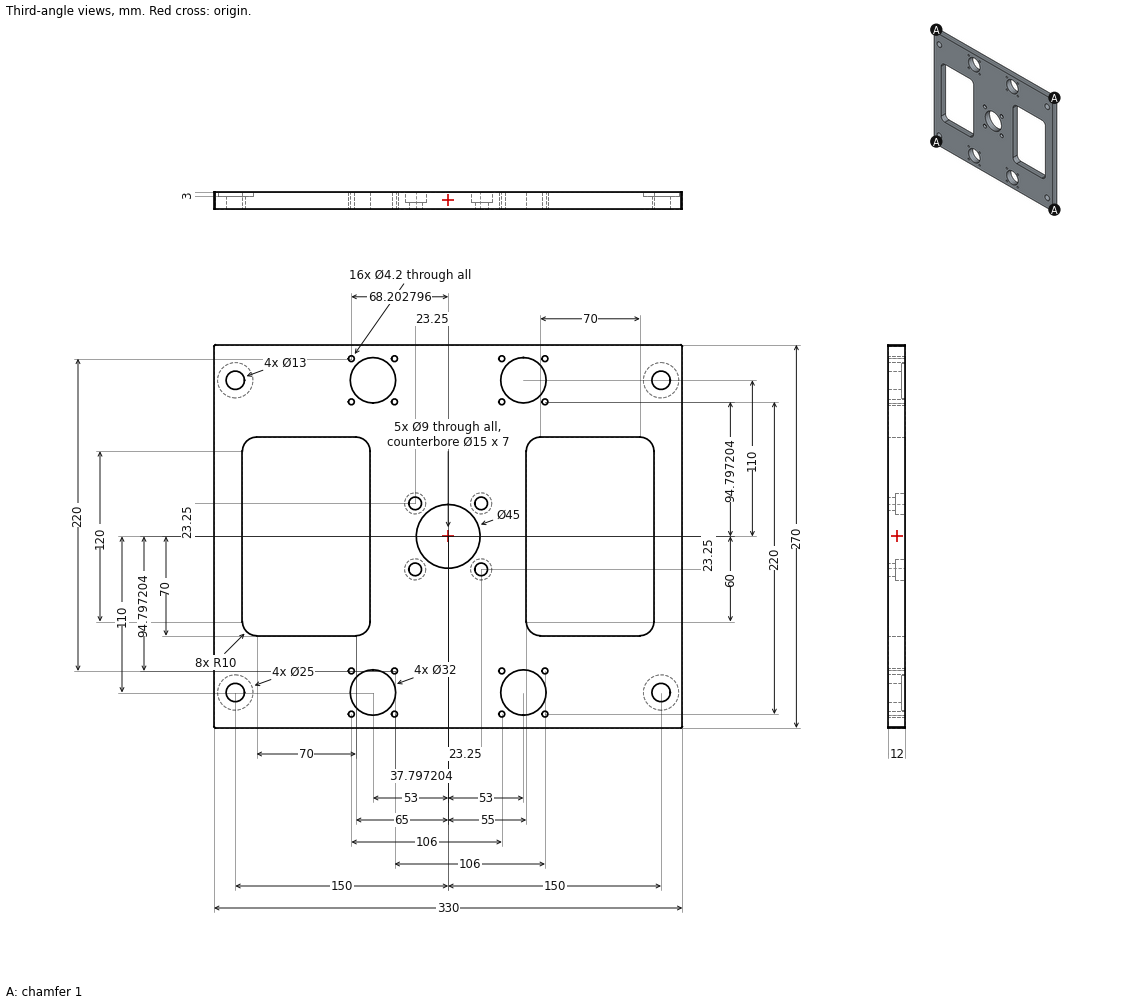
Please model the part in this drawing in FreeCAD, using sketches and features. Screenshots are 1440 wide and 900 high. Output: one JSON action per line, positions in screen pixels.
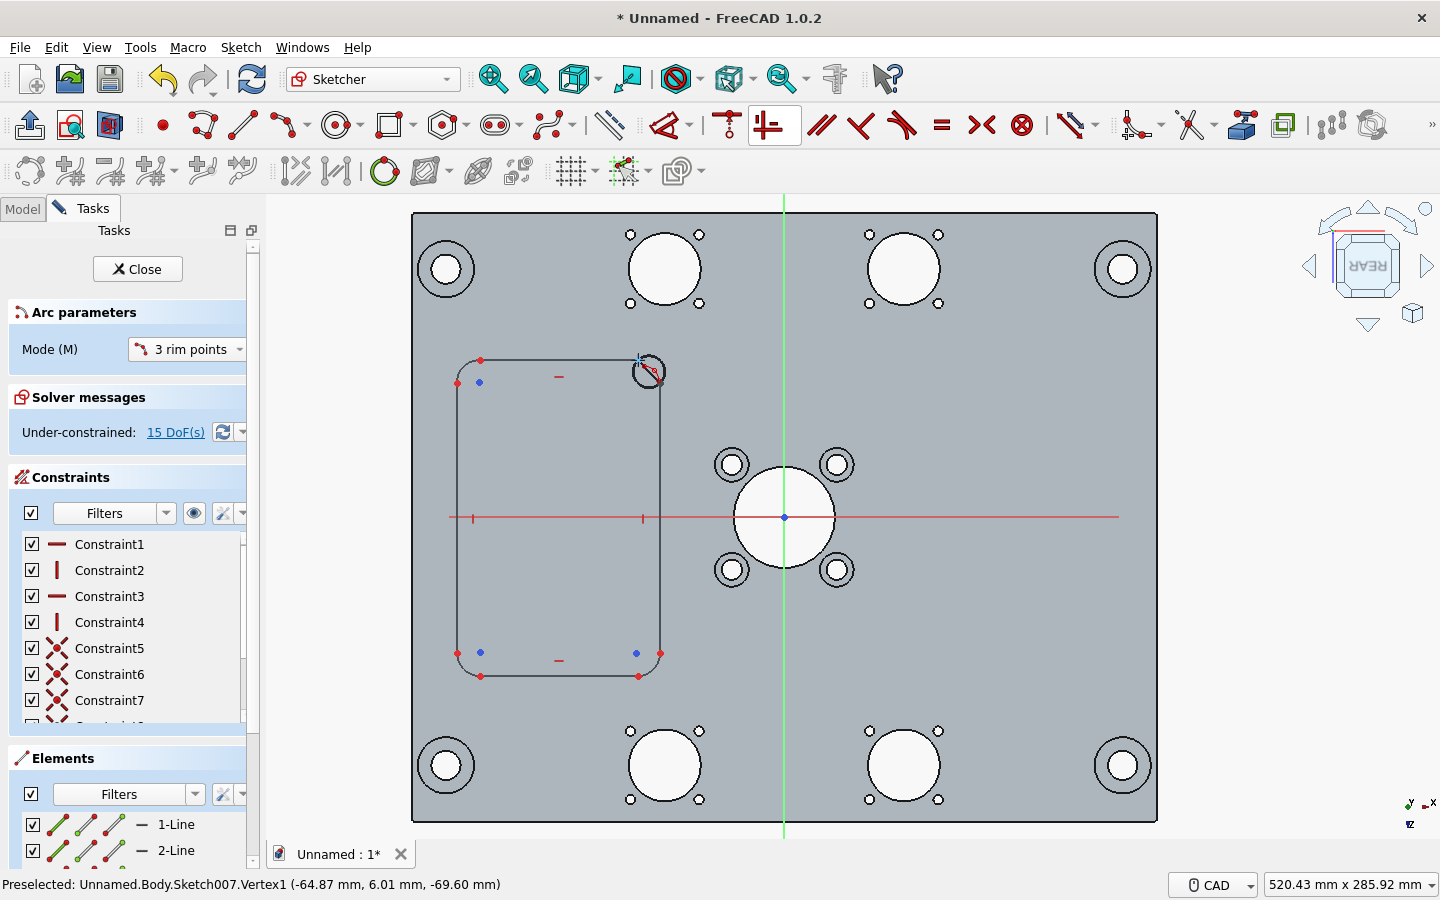
{"action": "scroll", "coordinate": [654, 366], "scroll_direction": "up", "scroll_amount": 5}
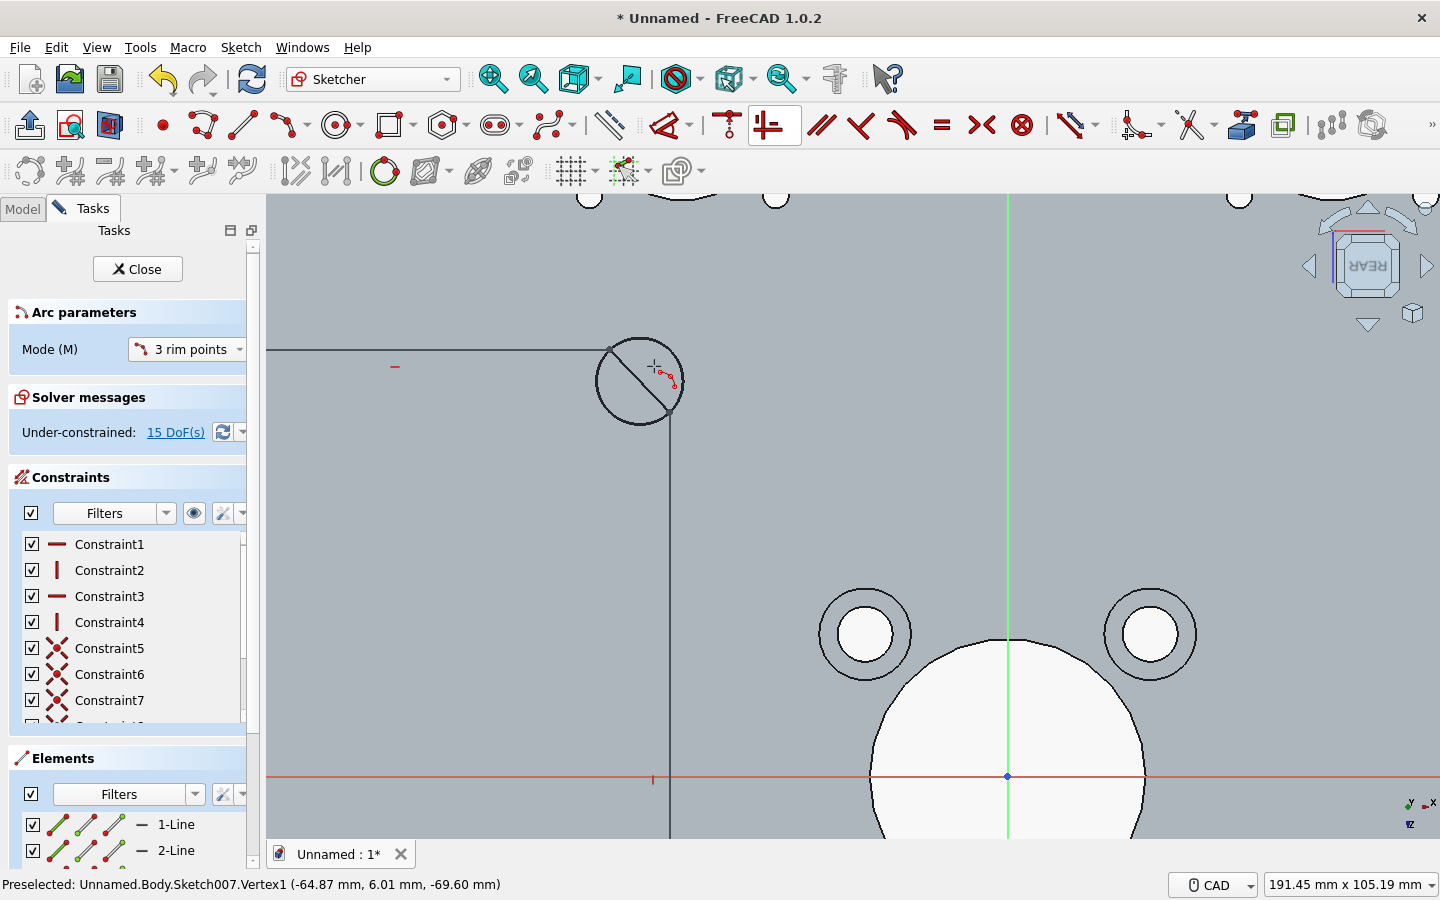
{"action": "left_click", "coordinate": [652, 365]}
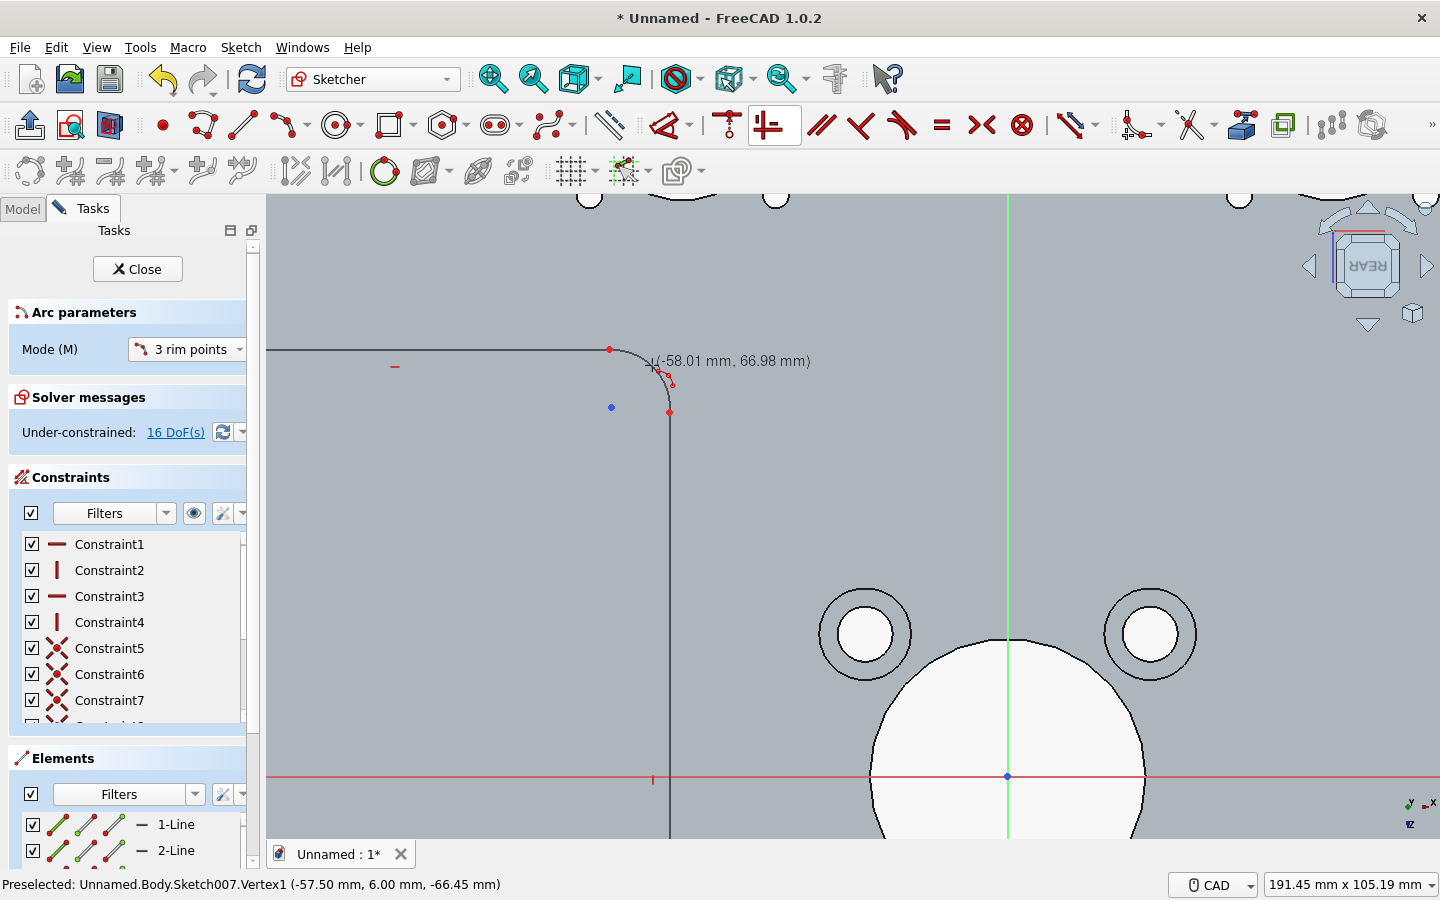
{"action": "key", "text": "g l"}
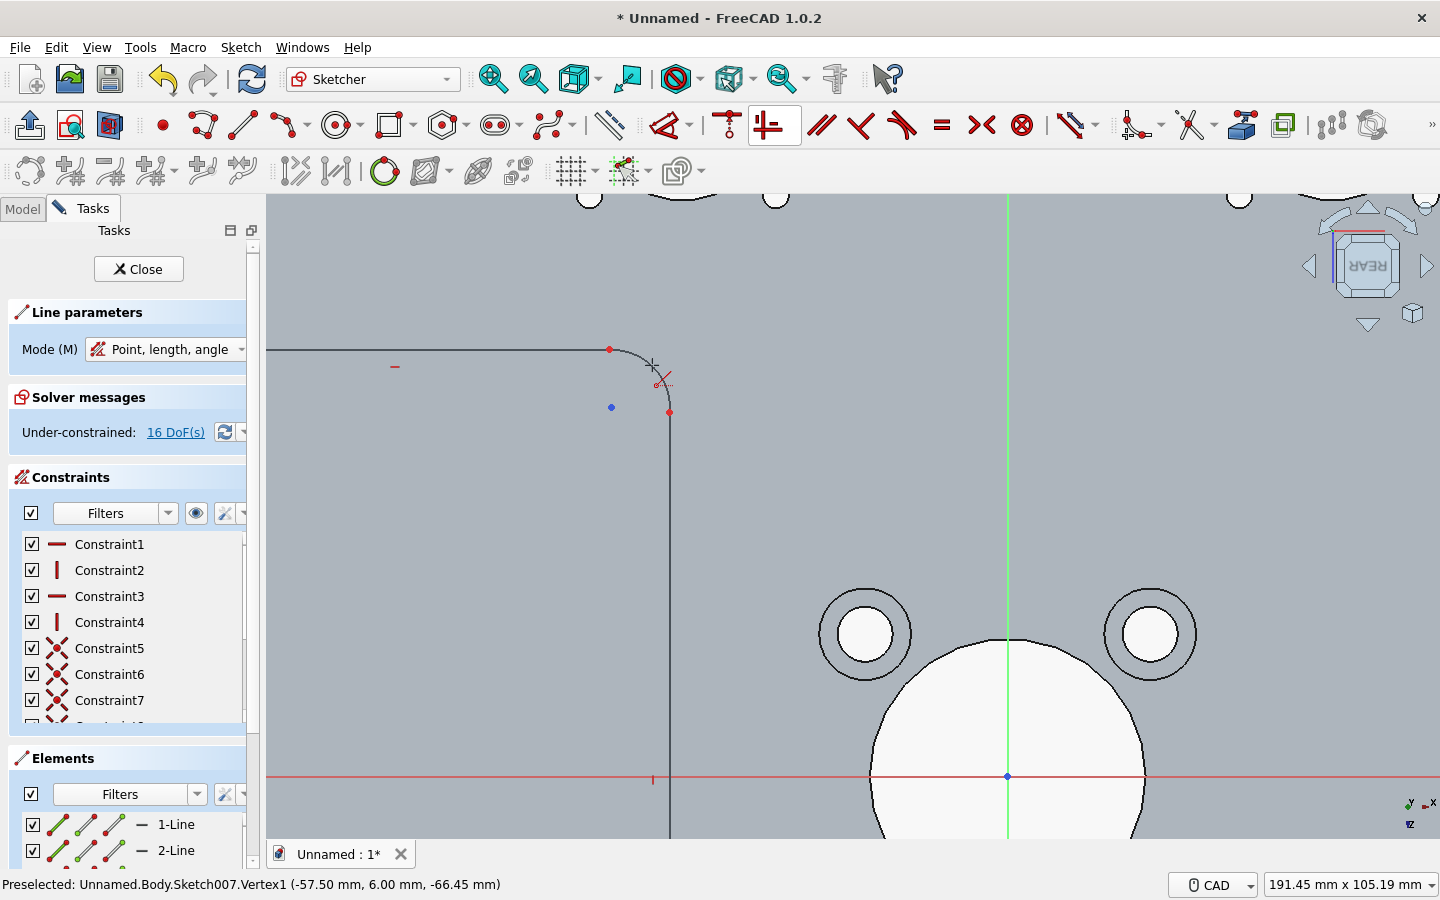
{"action": "scroll", "coordinate": [655, 365], "scroll_direction": "down", "scroll_amount": 5}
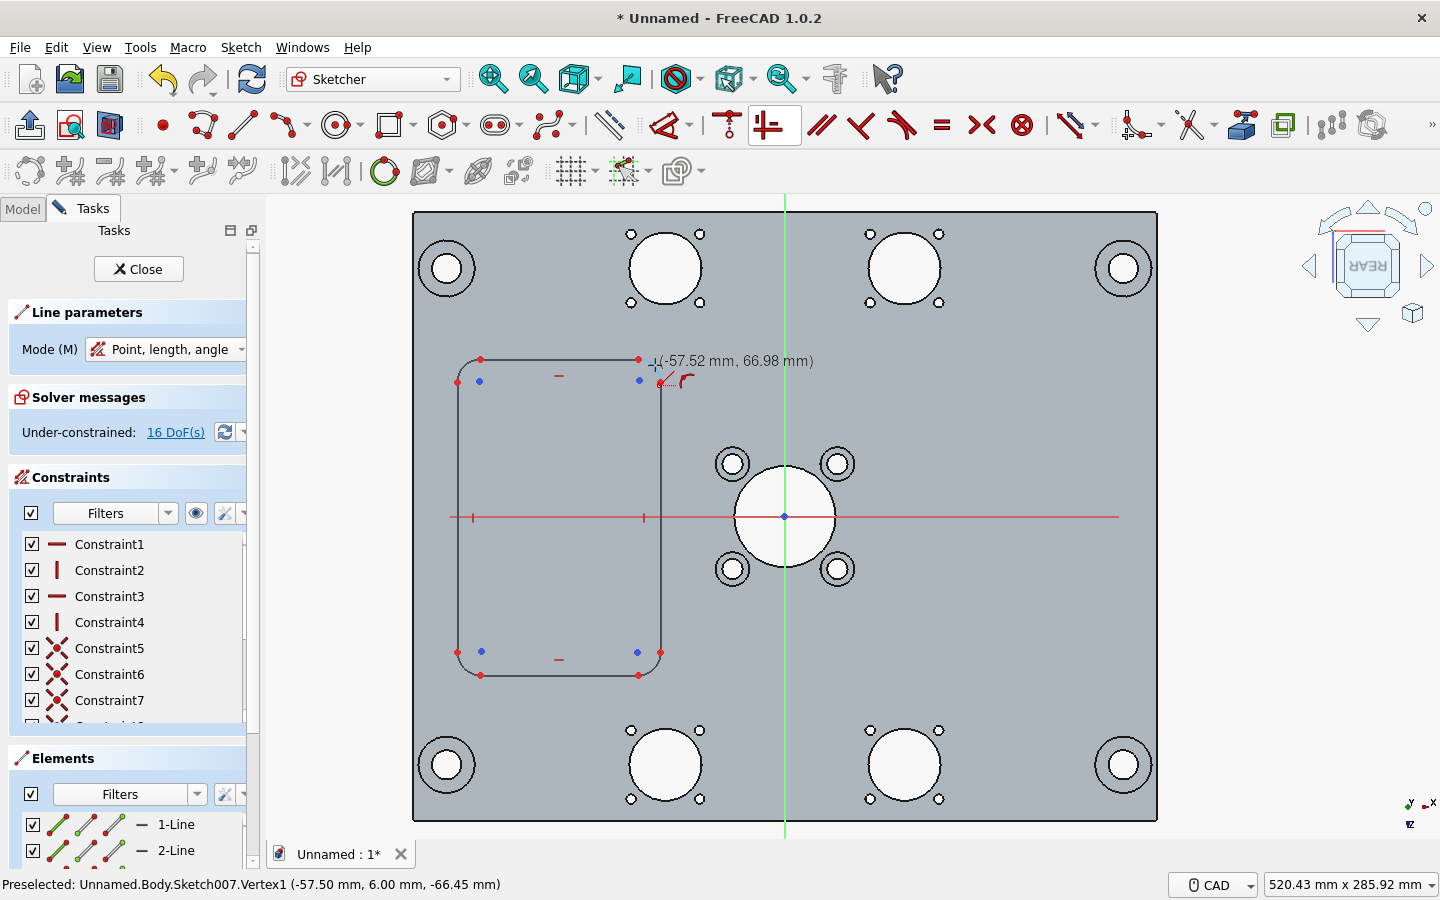
{"action": "left_click", "coordinate": [909, 381]}
{"action": "left_click", "coordinate": [909, 652]}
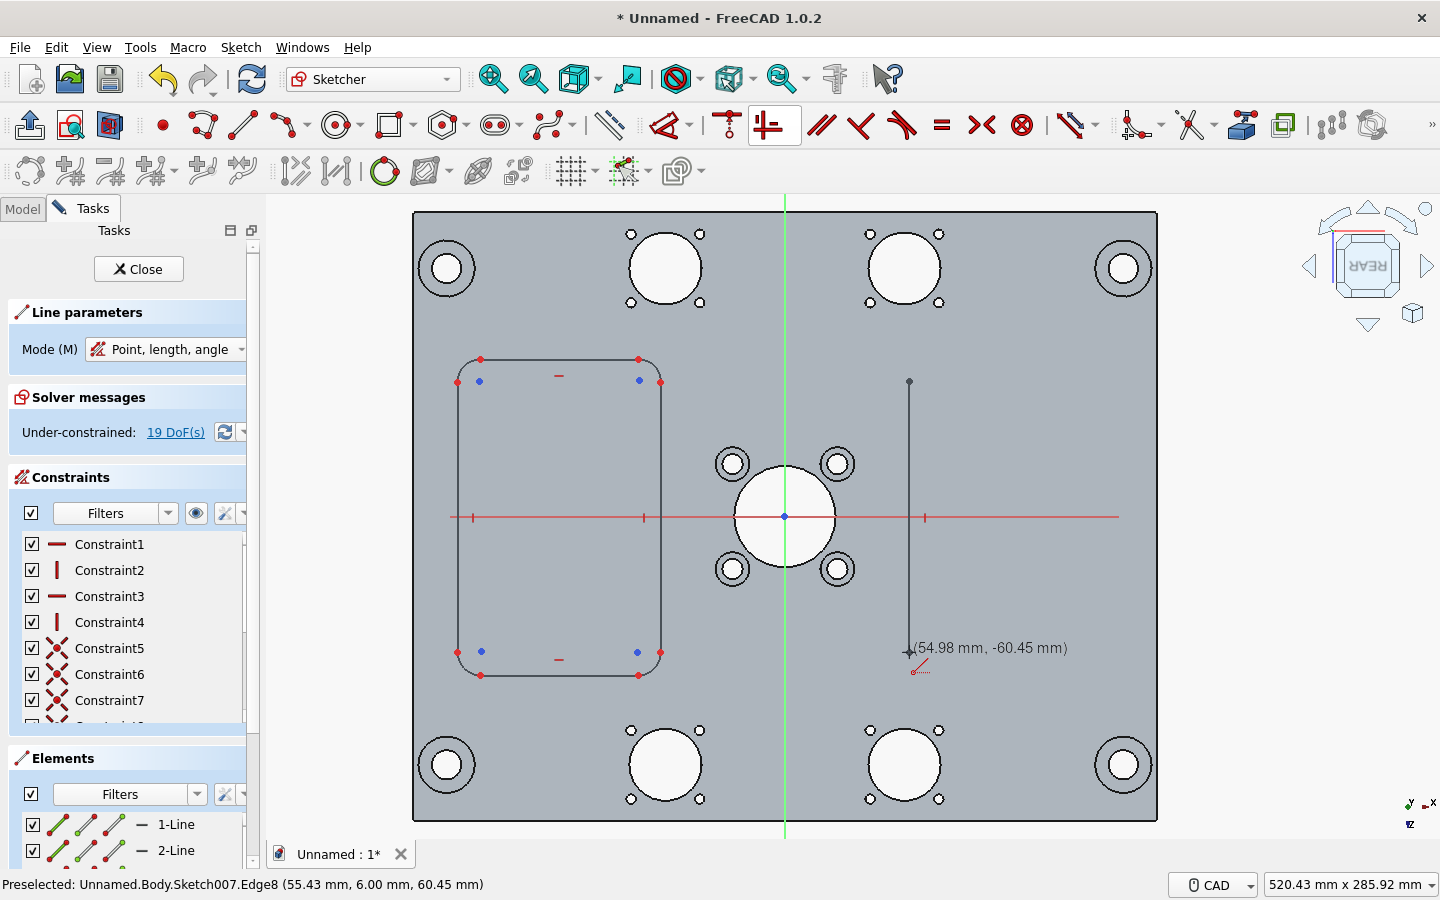
{"action": "left_click", "coordinate": [932, 675]}
{"action": "left_click", "coordinate": [1090, 675]}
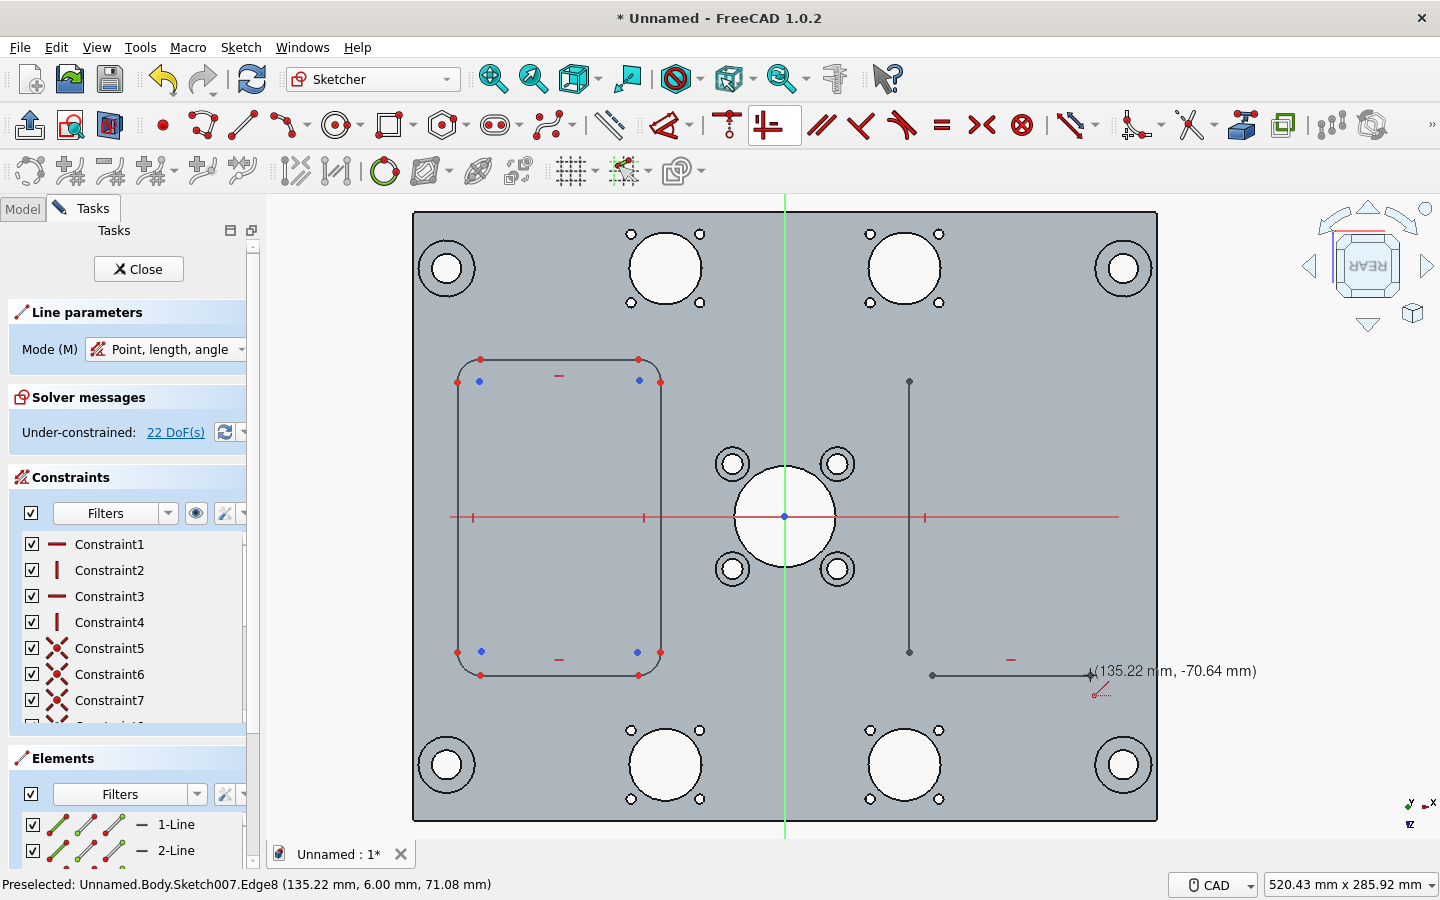
{"action": "left_click", "coordinate": [1112, 652]}
{"action": "left_click", "coordinate": [1112, 381]}